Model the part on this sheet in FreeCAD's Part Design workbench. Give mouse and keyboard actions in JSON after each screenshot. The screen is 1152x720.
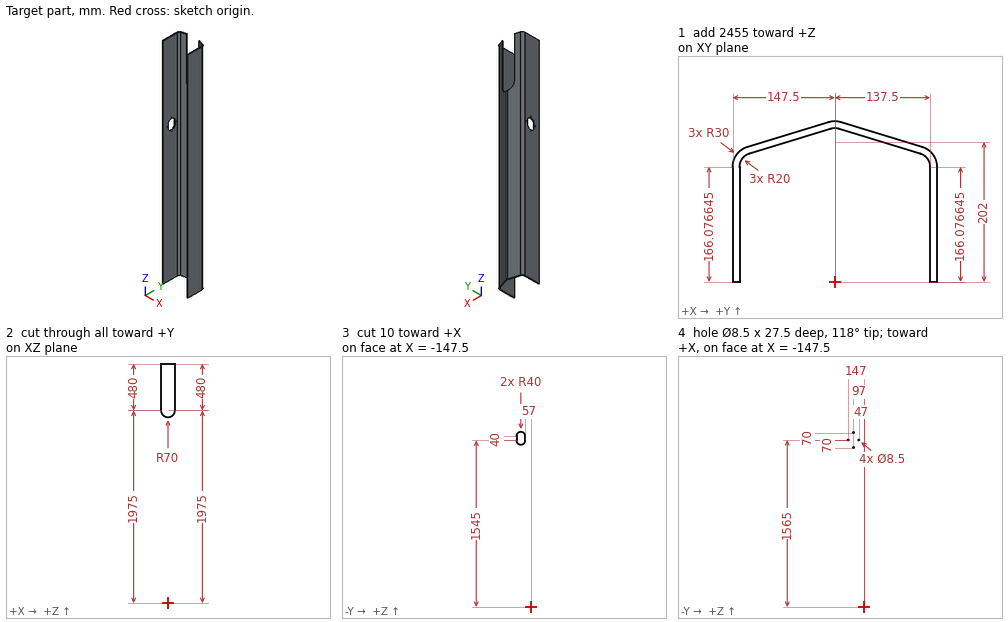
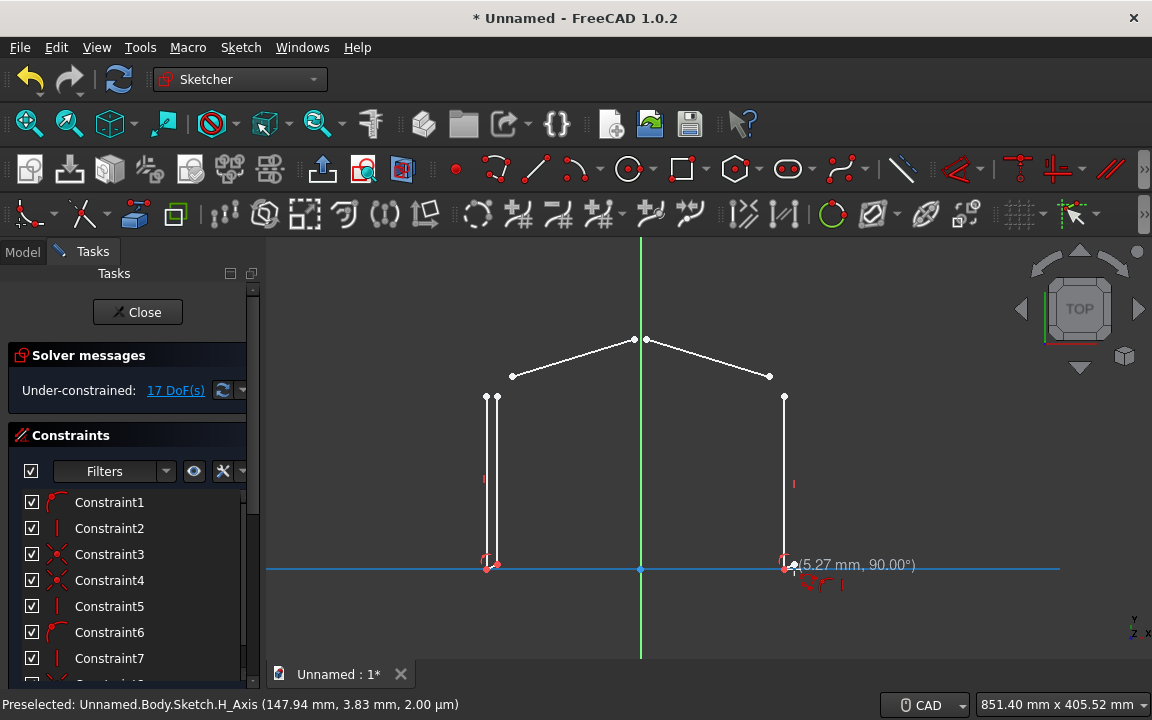
{"action": "scroll", "coordinate": [794, 396], "scroll_direction": "up", "scroll_amount": 3}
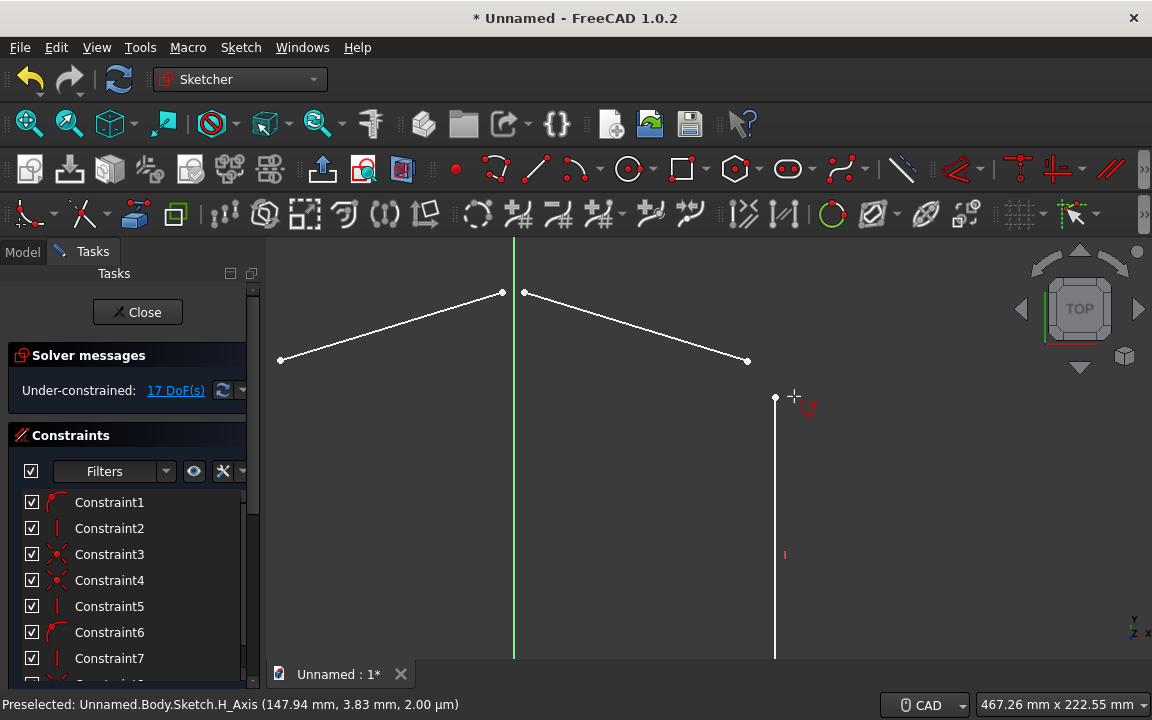
{"action": "left_click", "coordinate": [794, 396]}
{"action": "right_click", "coordinate": [794, 396]}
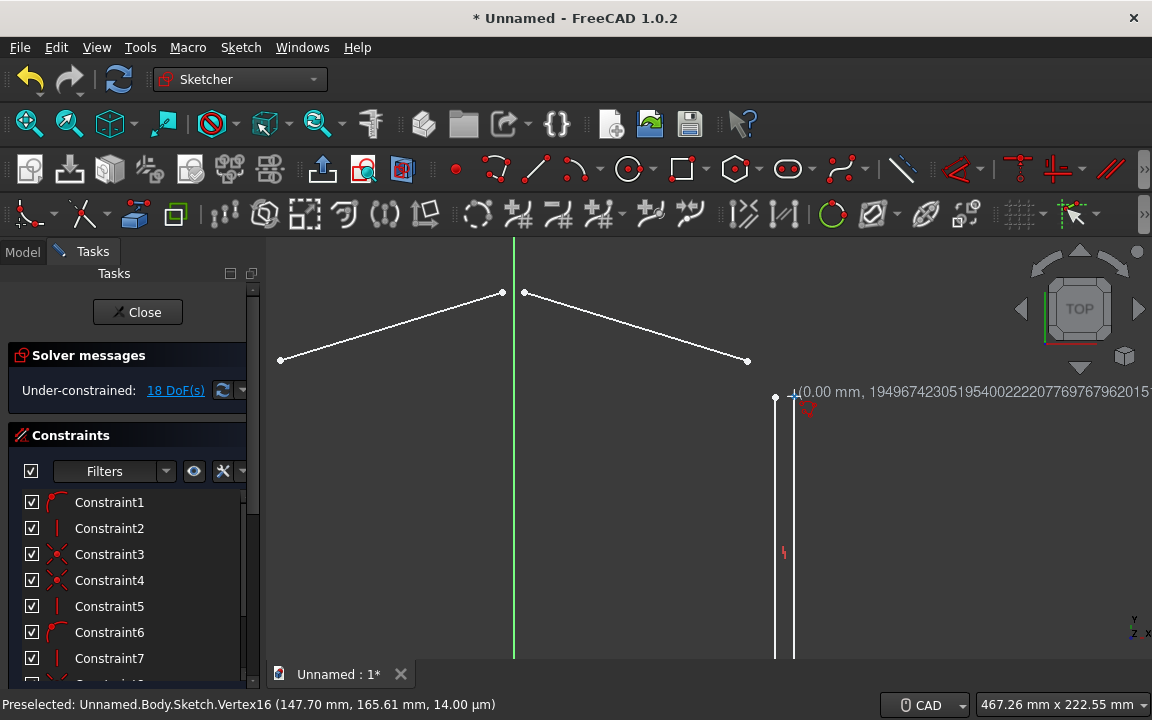
{"action": "left_click", "coordinate": [536, 170]}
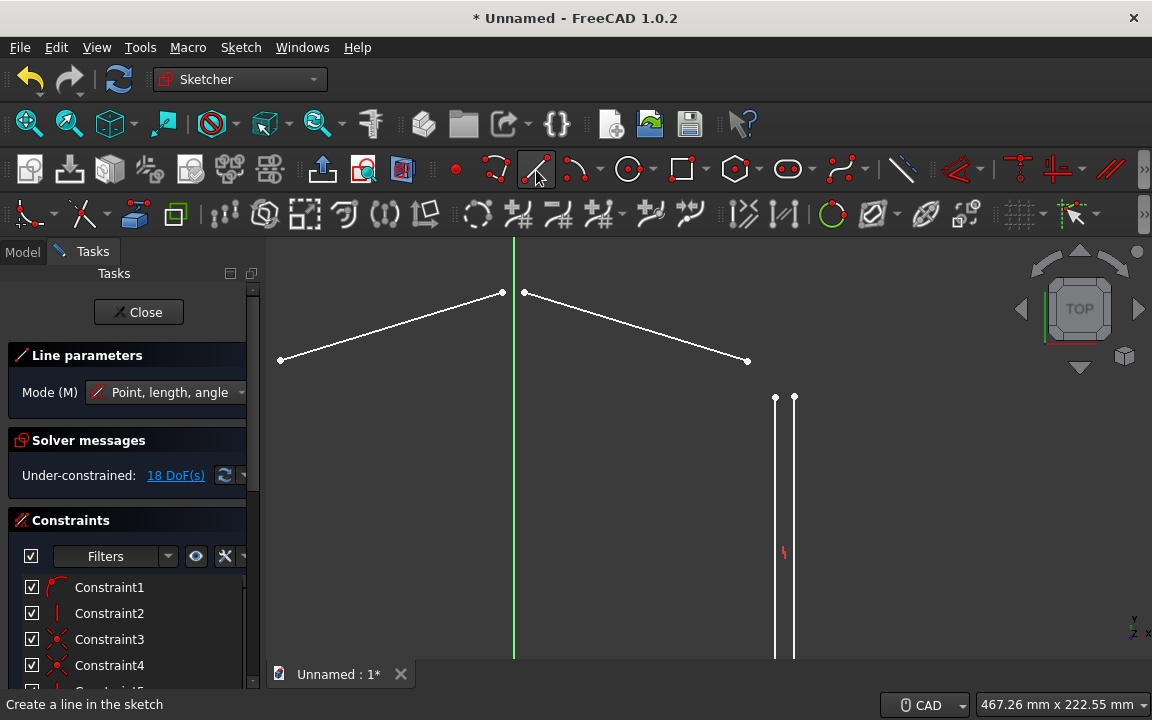
{"action": "left_click", "coordinate": [753, 342]}
{"action": "left_click", "coordinate": [531, 274]}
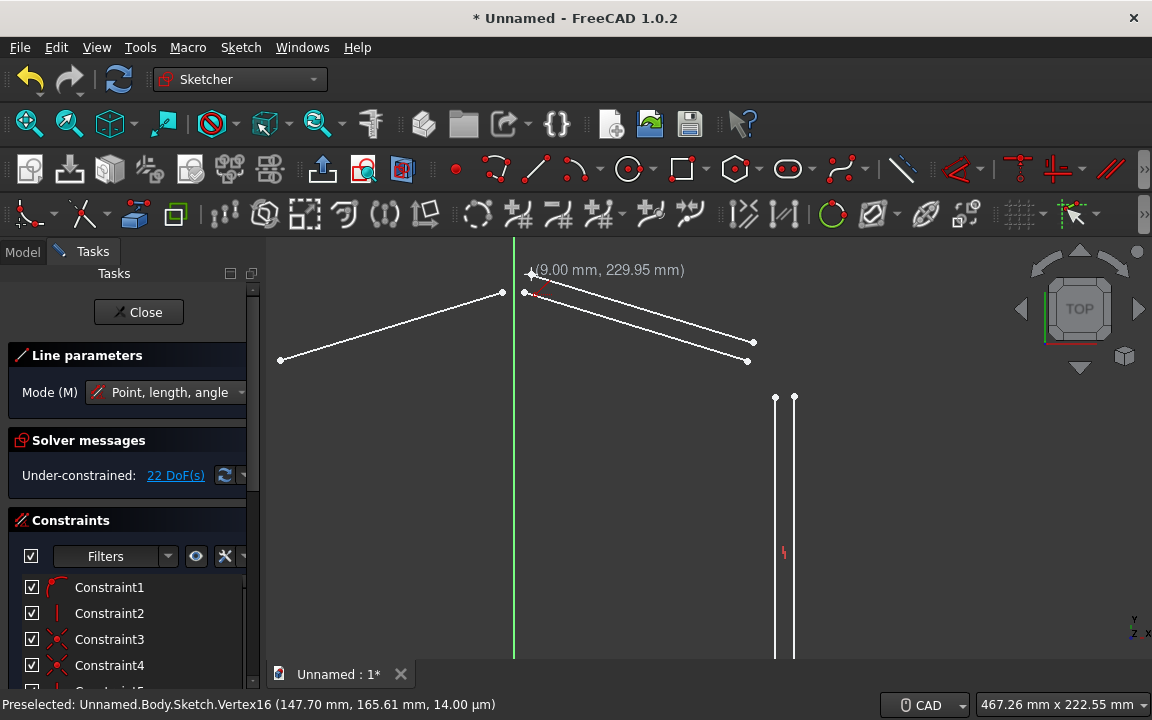
{"action": "left_click", "coordinate": [497, 274]}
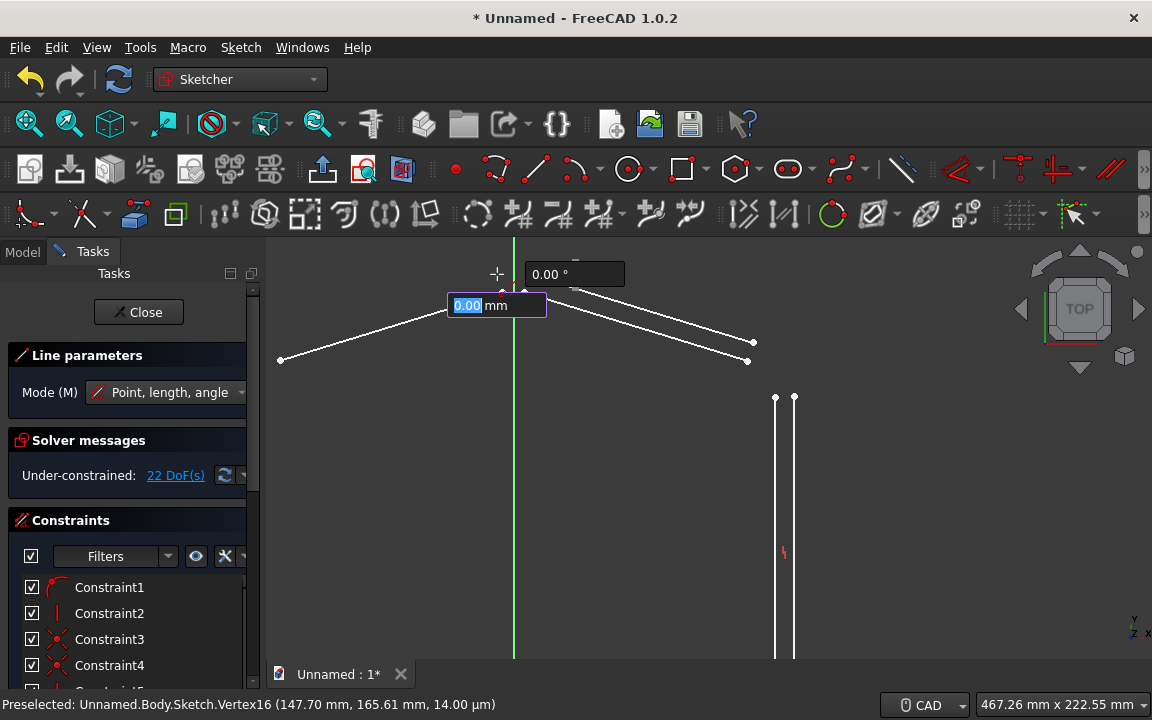
{"action": "scroll", "coordinate": [794, 396], "scroll_direction": "down", "scroll_amount": 3}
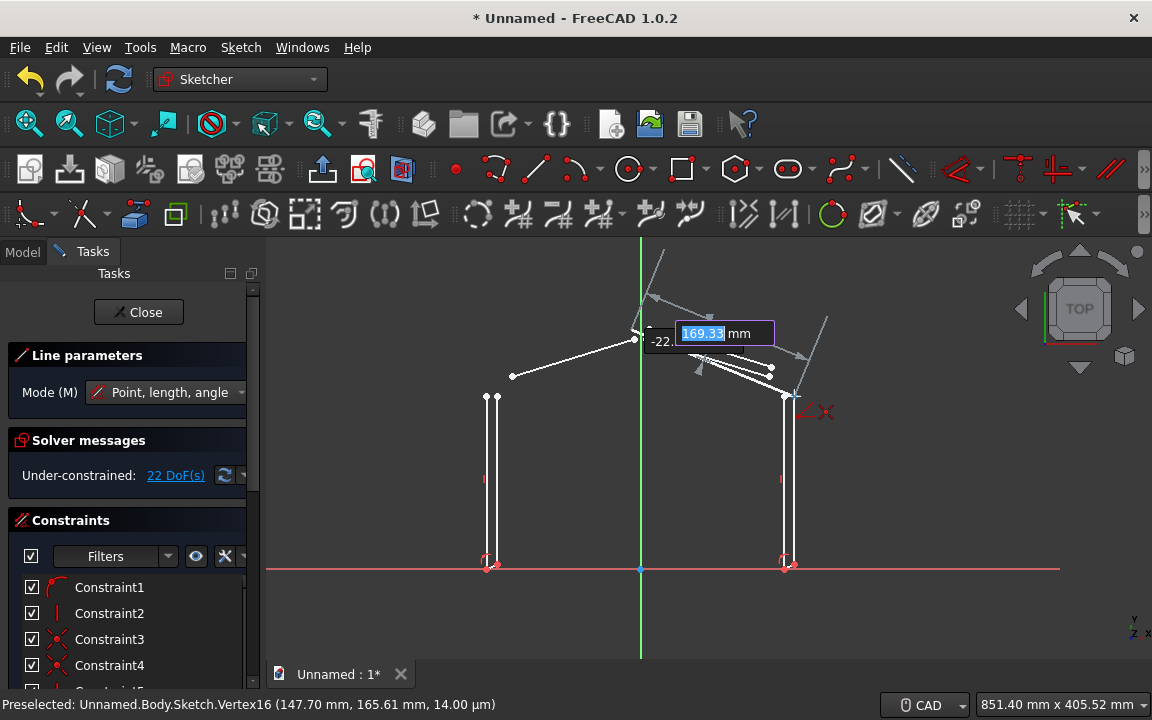
{"action": "scroll", "coordinate": [509, 366], "scroll_direction": "up", "scroll_amount": 3}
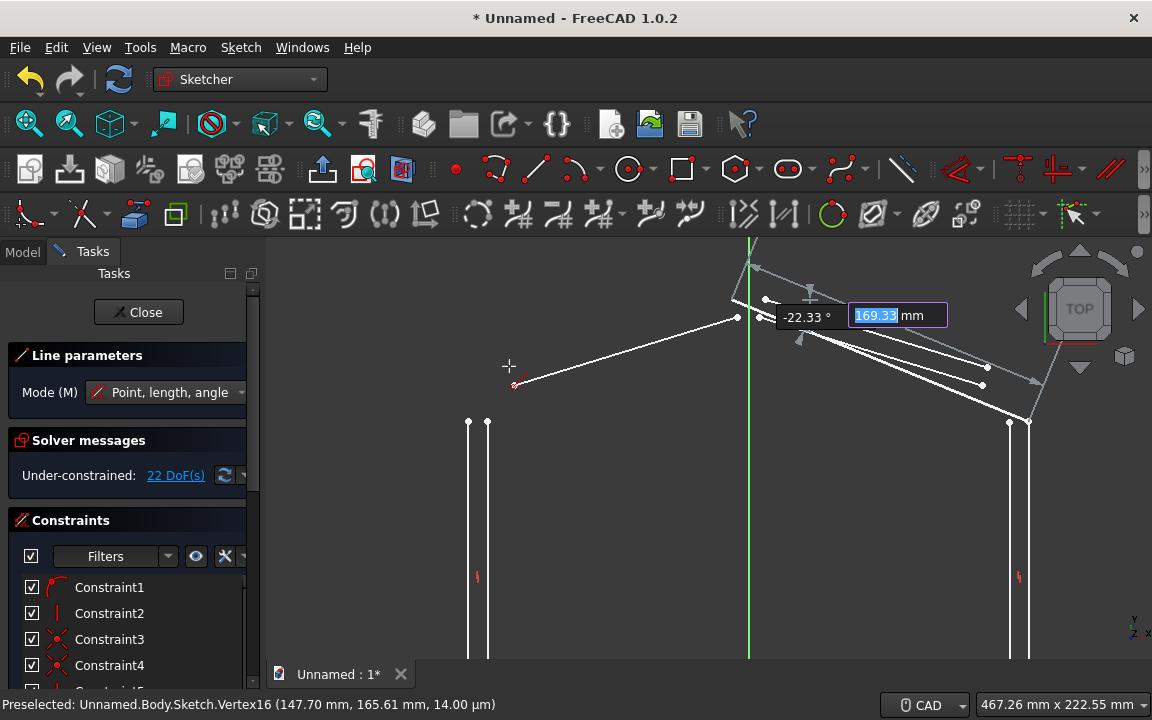
{"action": "left_click", "coordinate": [509, 366]}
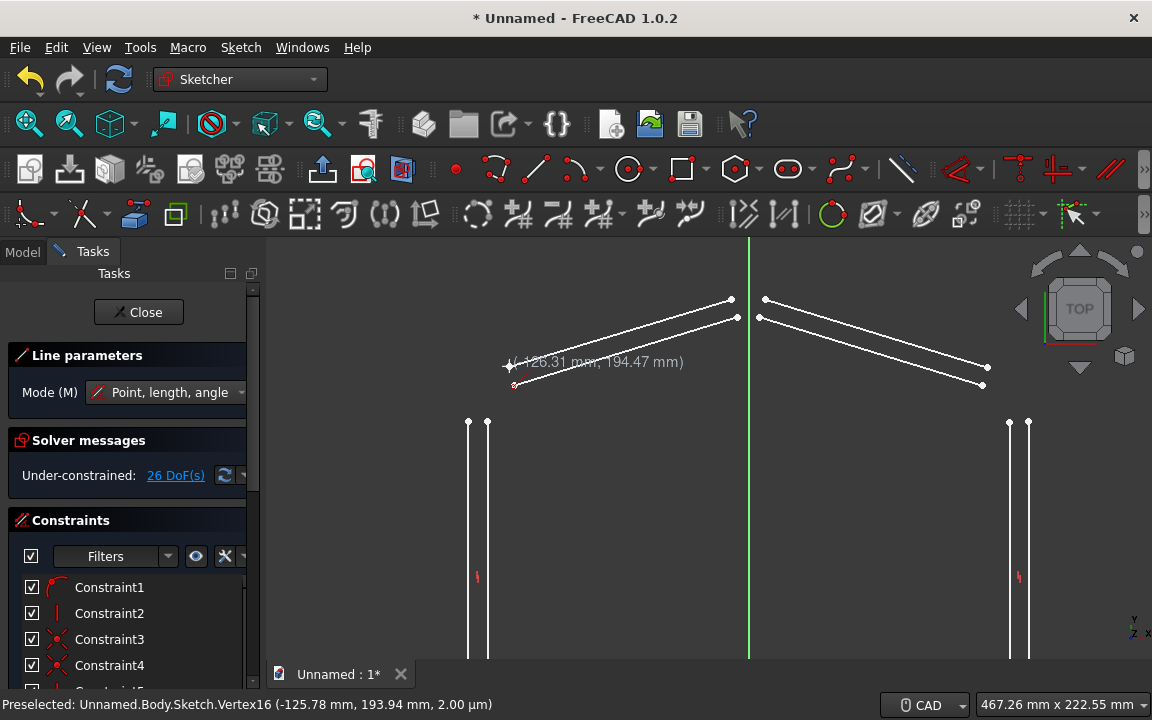
{"action": "left_click", "coordinate": [602, 170]}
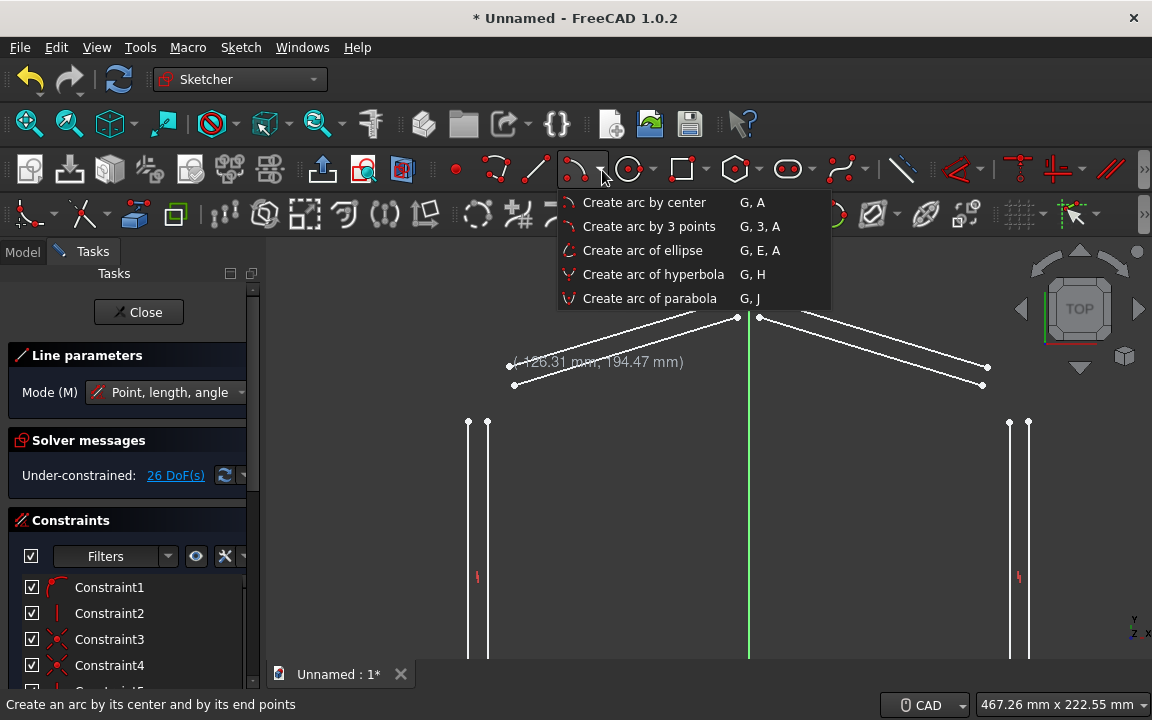
{"action": "left_click", "coordinate": [694, 226]}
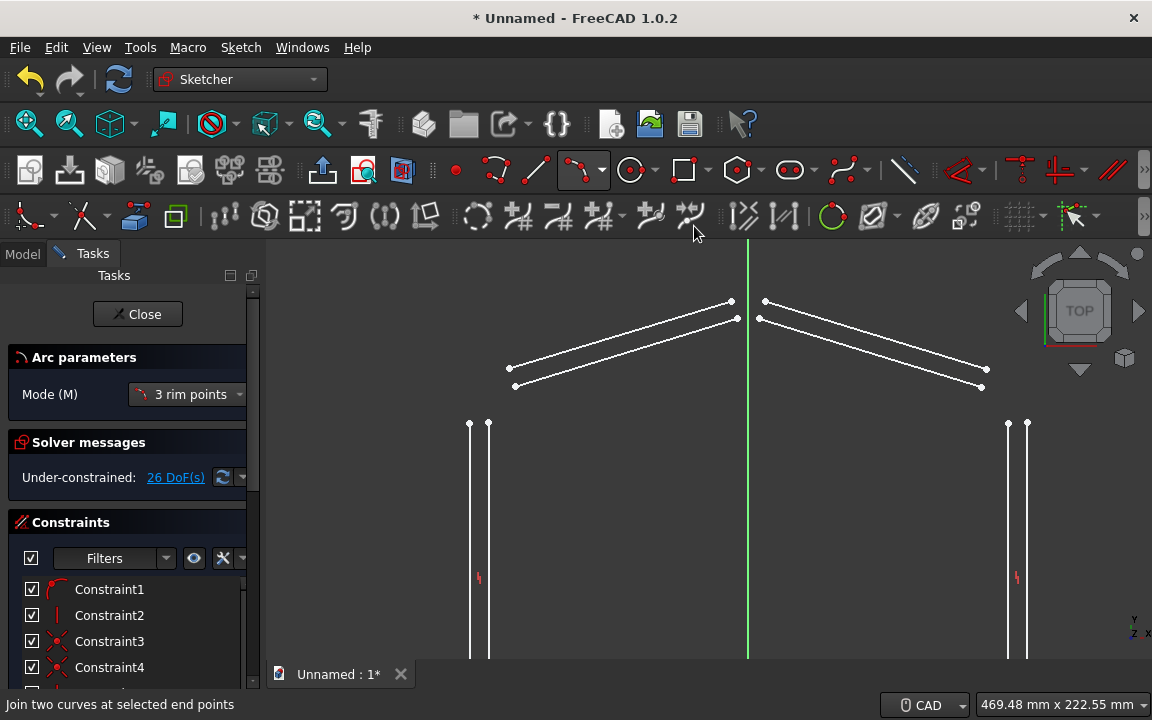
{"action": "left_click", "coordinate": [489, 423]}
{"action": "left_click", "coordinate": [516, 387]}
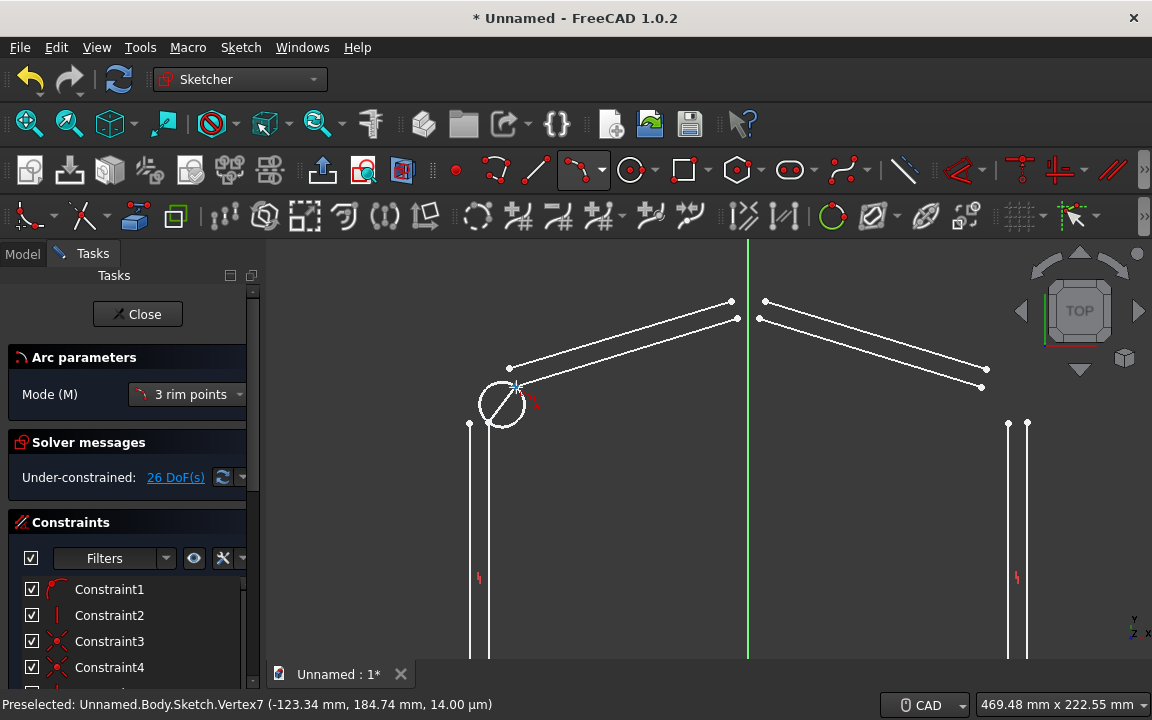
{"action": "scroll", "coordinate": [496, 400], "scroll_direction": "up", "scroll_amount": 4}